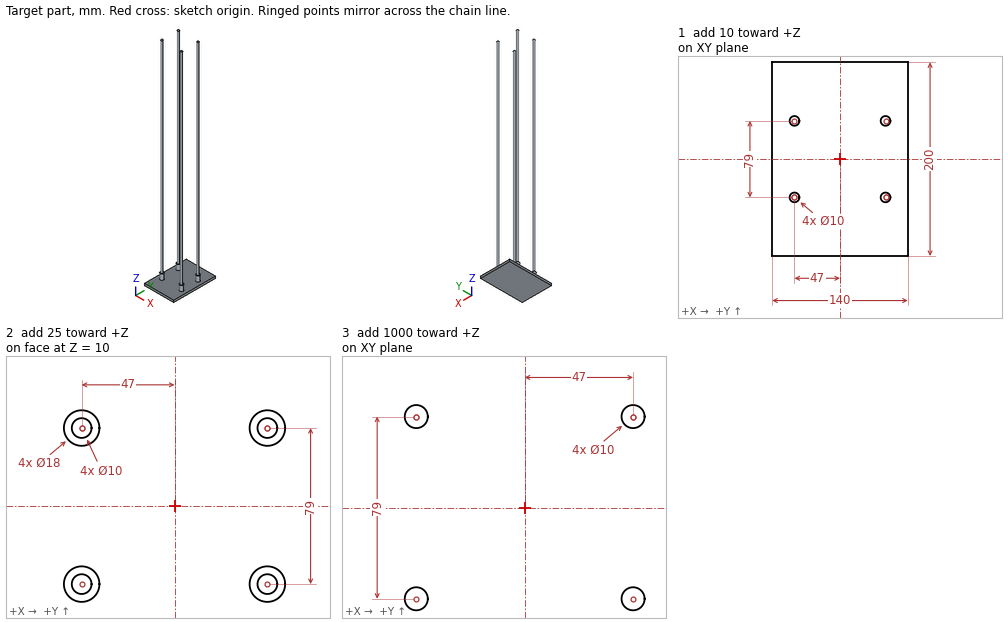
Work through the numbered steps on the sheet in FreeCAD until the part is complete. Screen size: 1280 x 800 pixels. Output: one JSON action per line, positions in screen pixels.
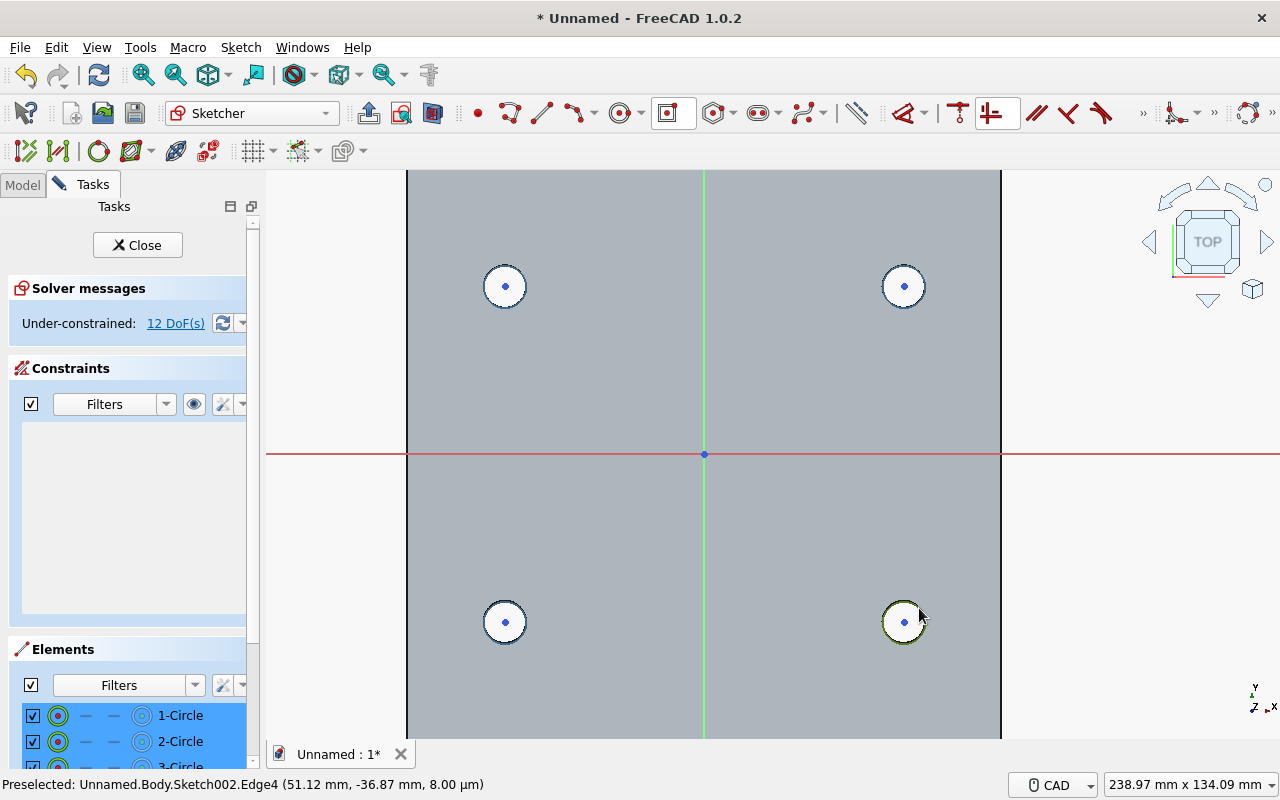
{"action": "key", "text": "e"}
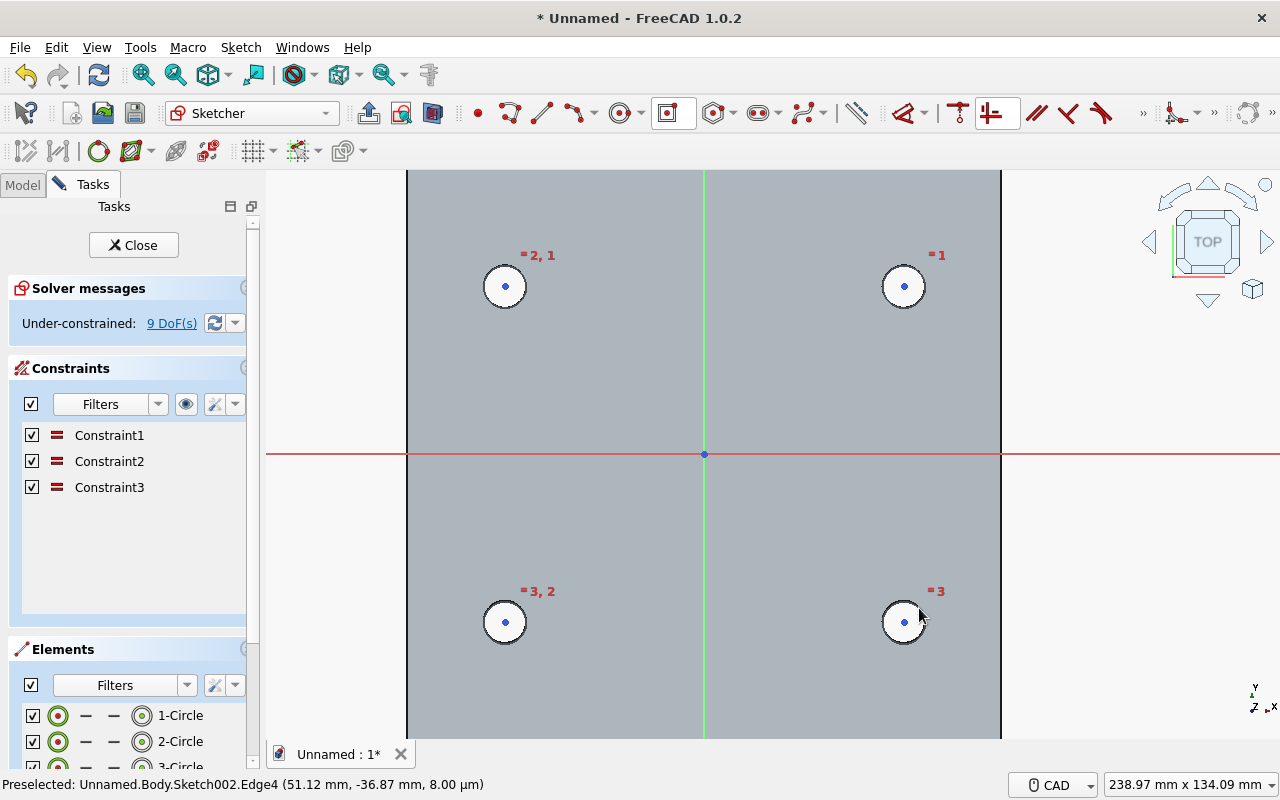
{"action": "left_click", "coordinate": [904, 287]}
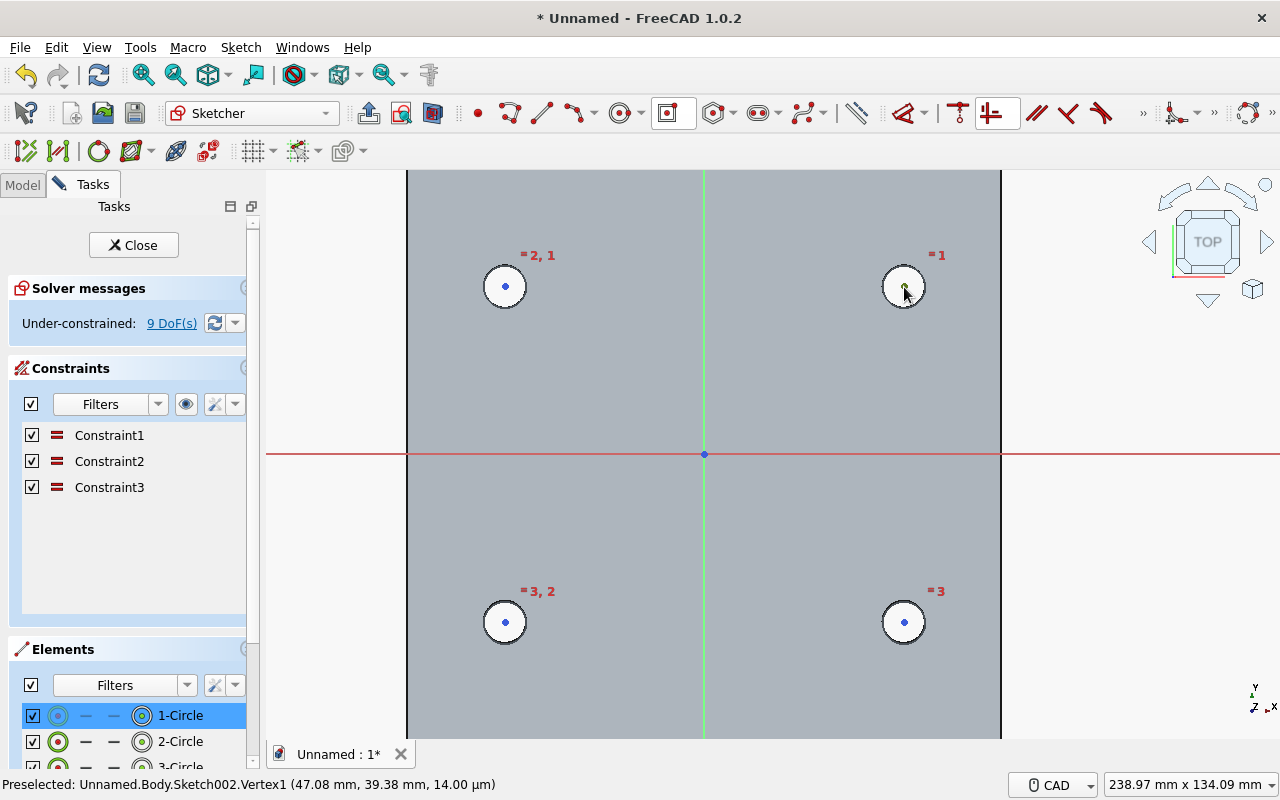
{"action": "left_click", "coordinate": [505, 287]}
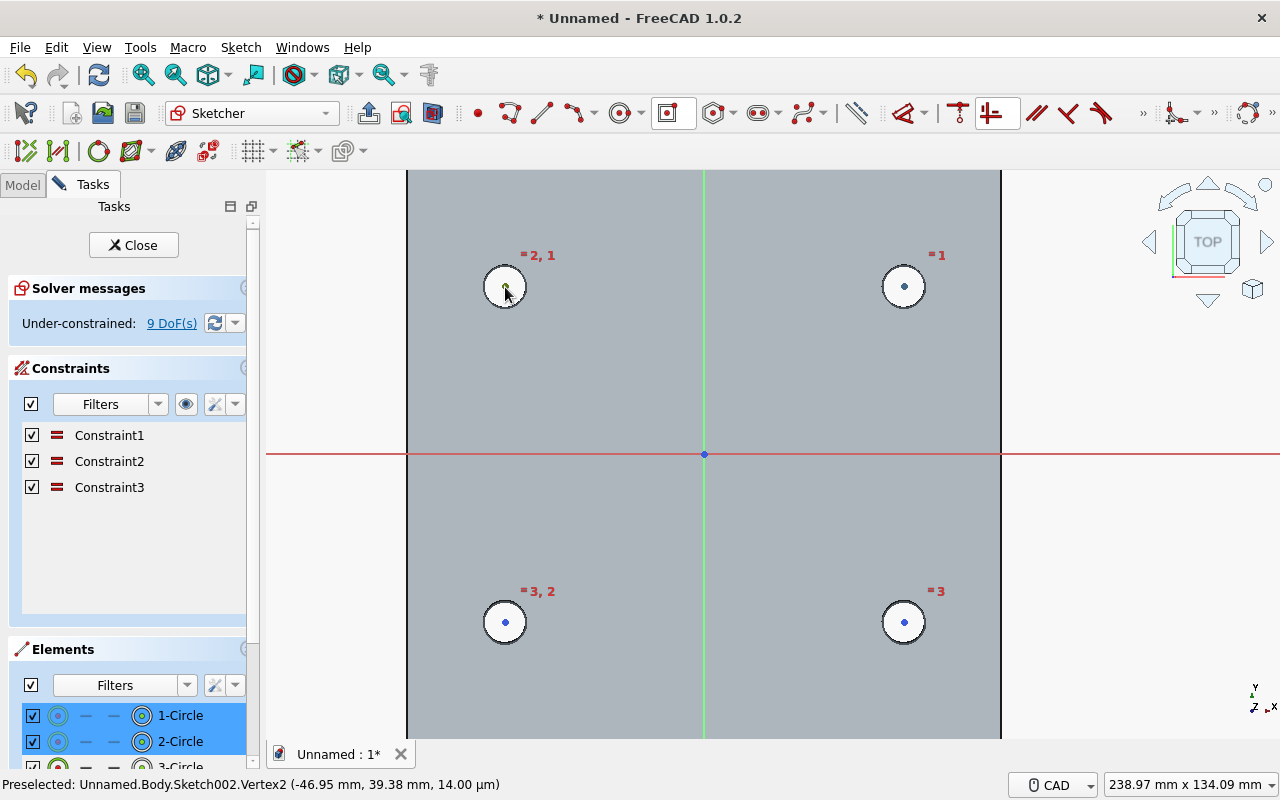
{"action": "left_click", "coordinate": [704, 674]}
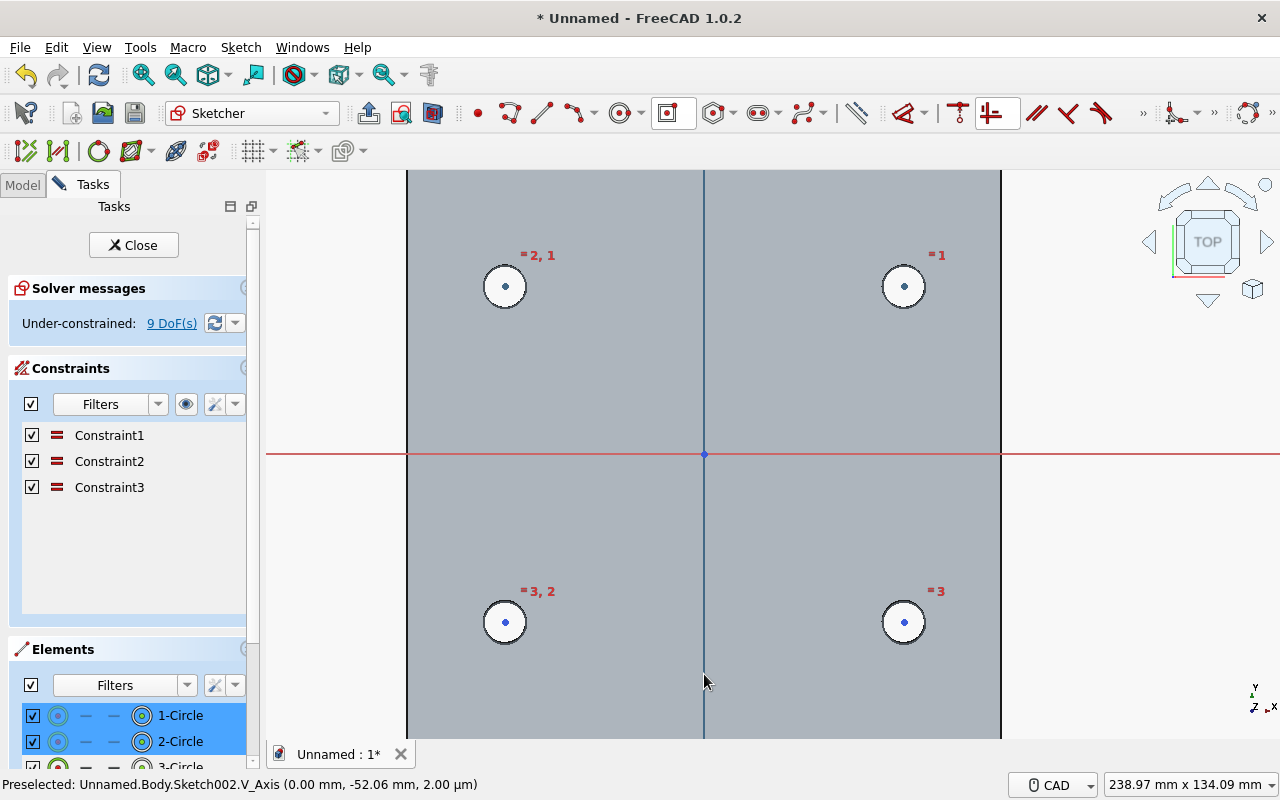
{"action": "key", "text": "s"}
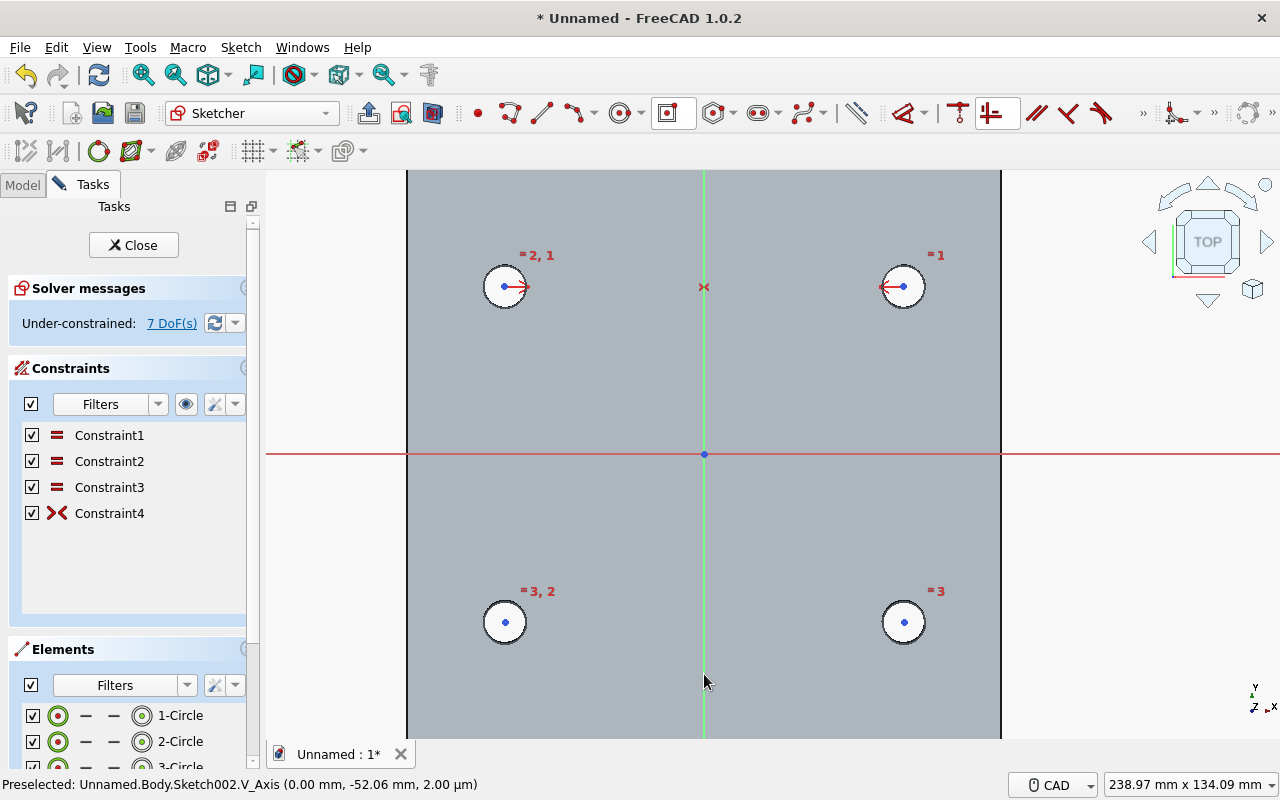
{"action": "left_click", "coordinate": [505, 287]}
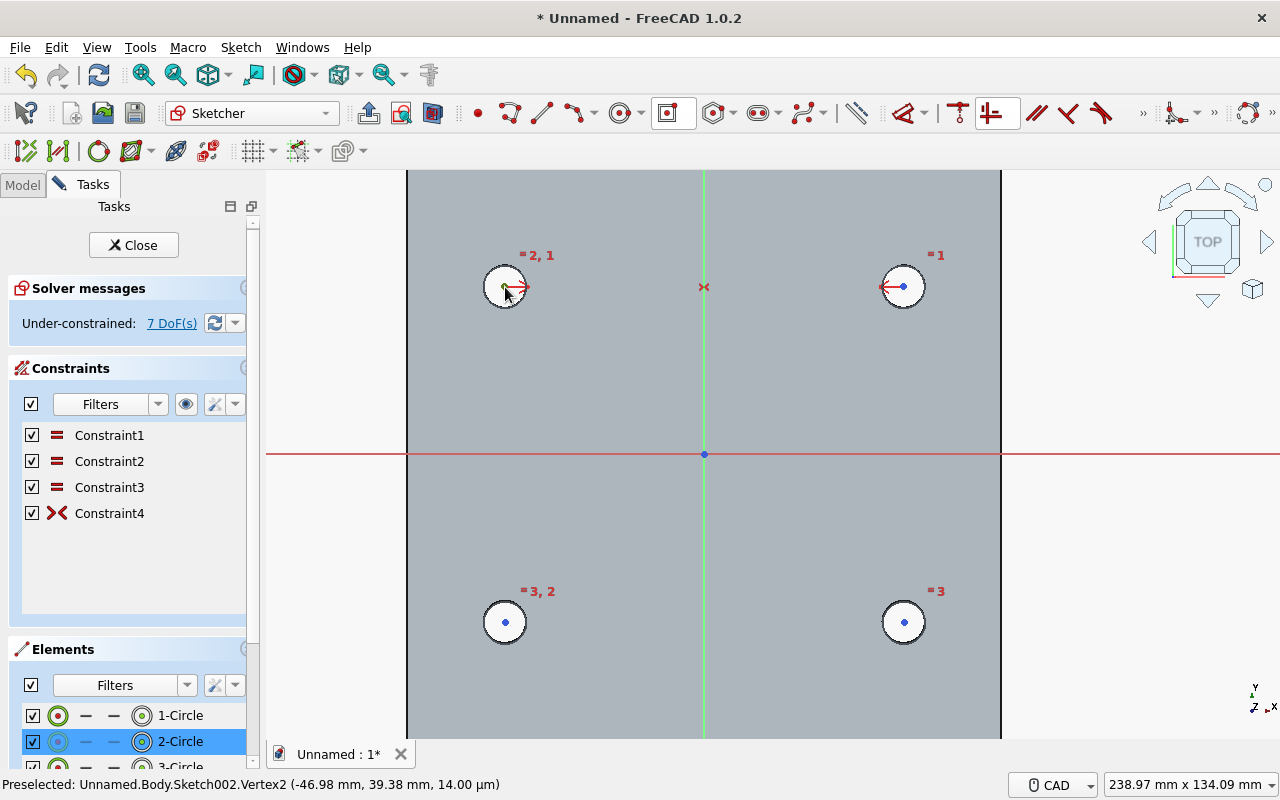
{"action": "left_click", "coordinate": [505, 623]}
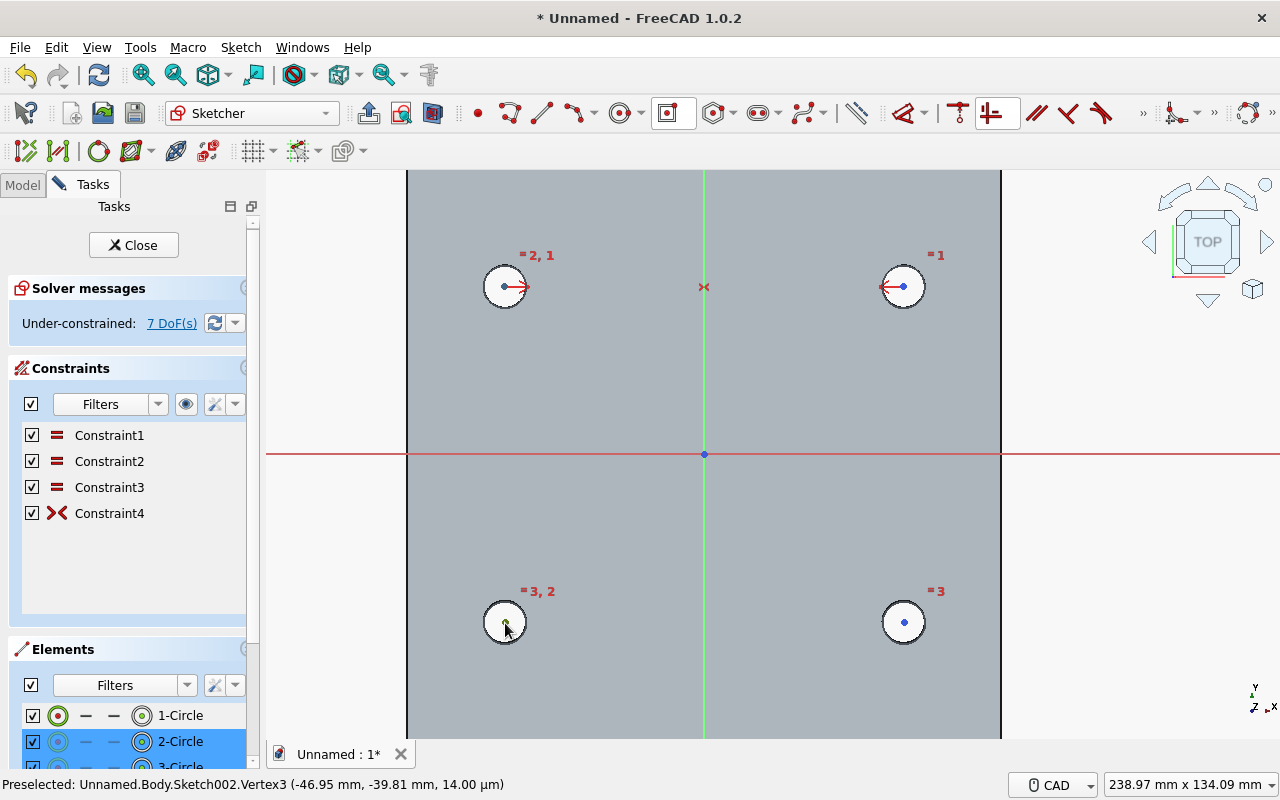
{"action": "left_click", "coordinate": [353, 454]}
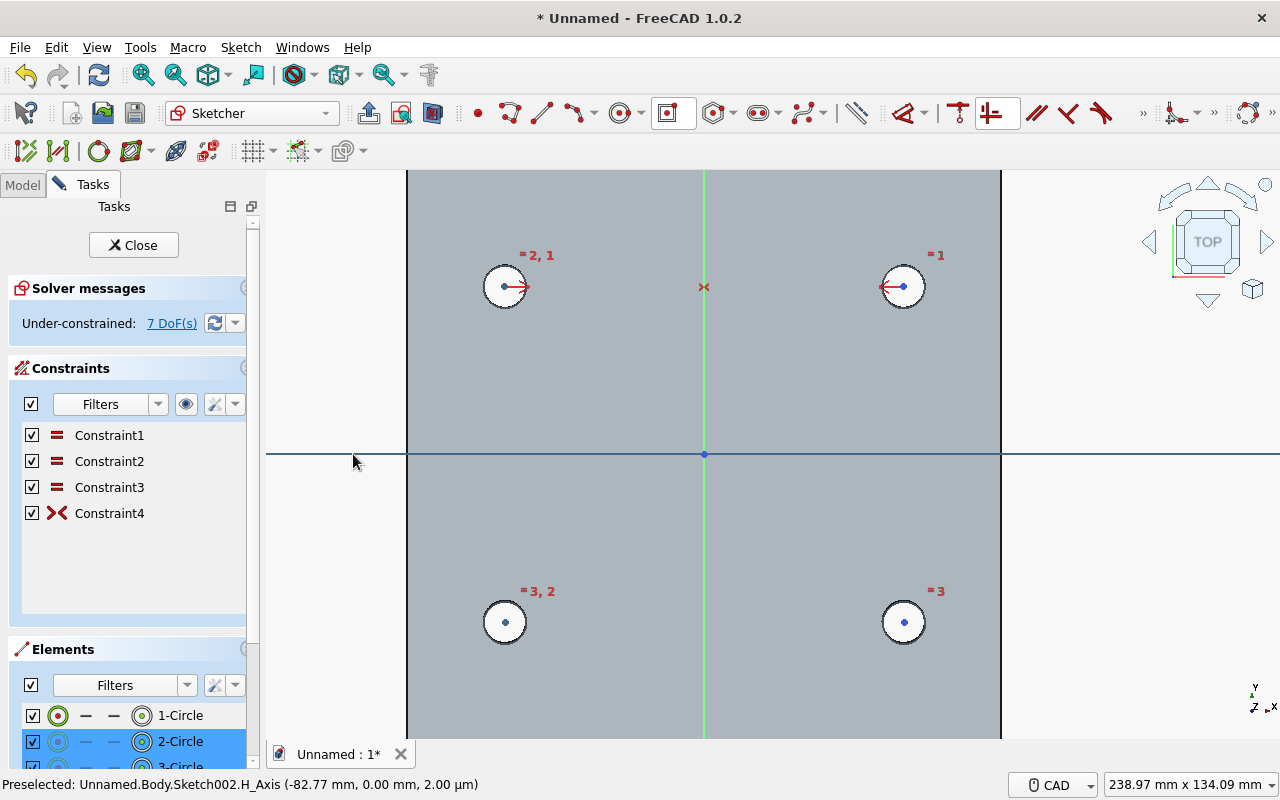
{"action": "key", "text": "s"}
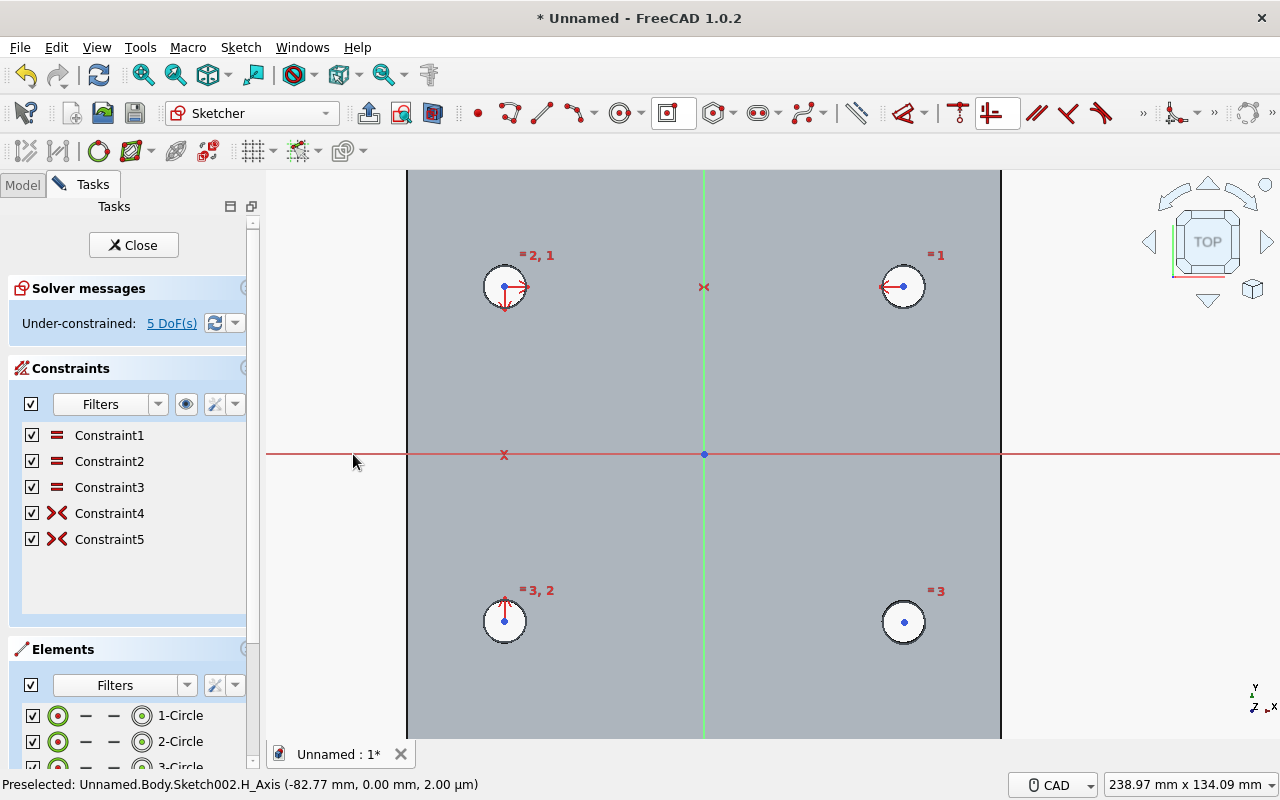
{"action": "left_click", "coordinate": [904, 287]}